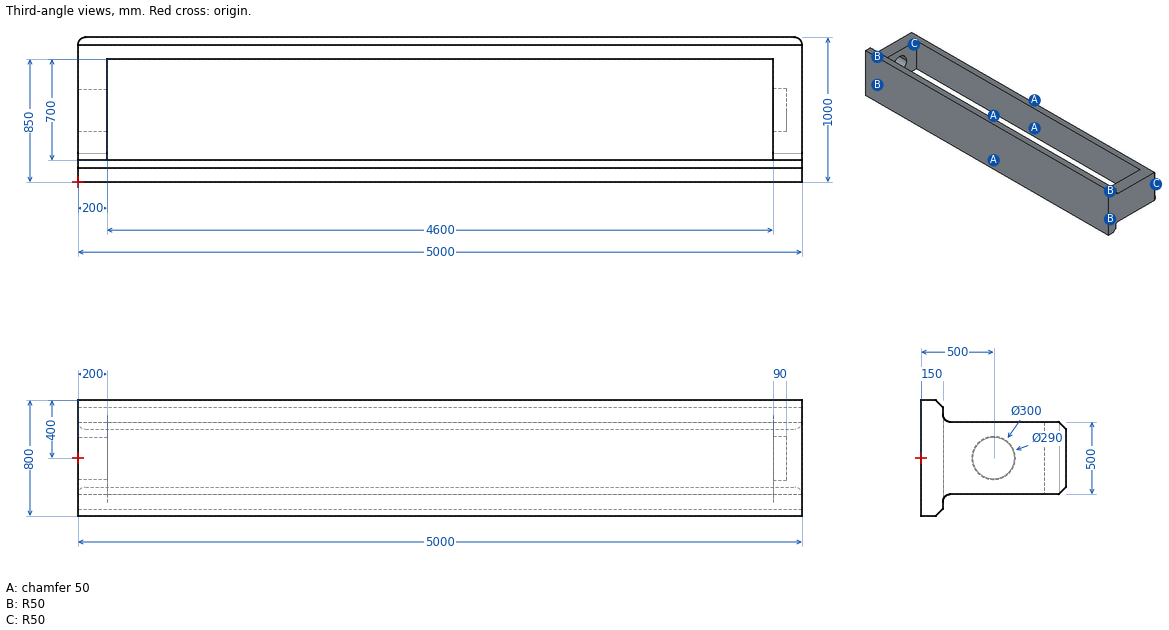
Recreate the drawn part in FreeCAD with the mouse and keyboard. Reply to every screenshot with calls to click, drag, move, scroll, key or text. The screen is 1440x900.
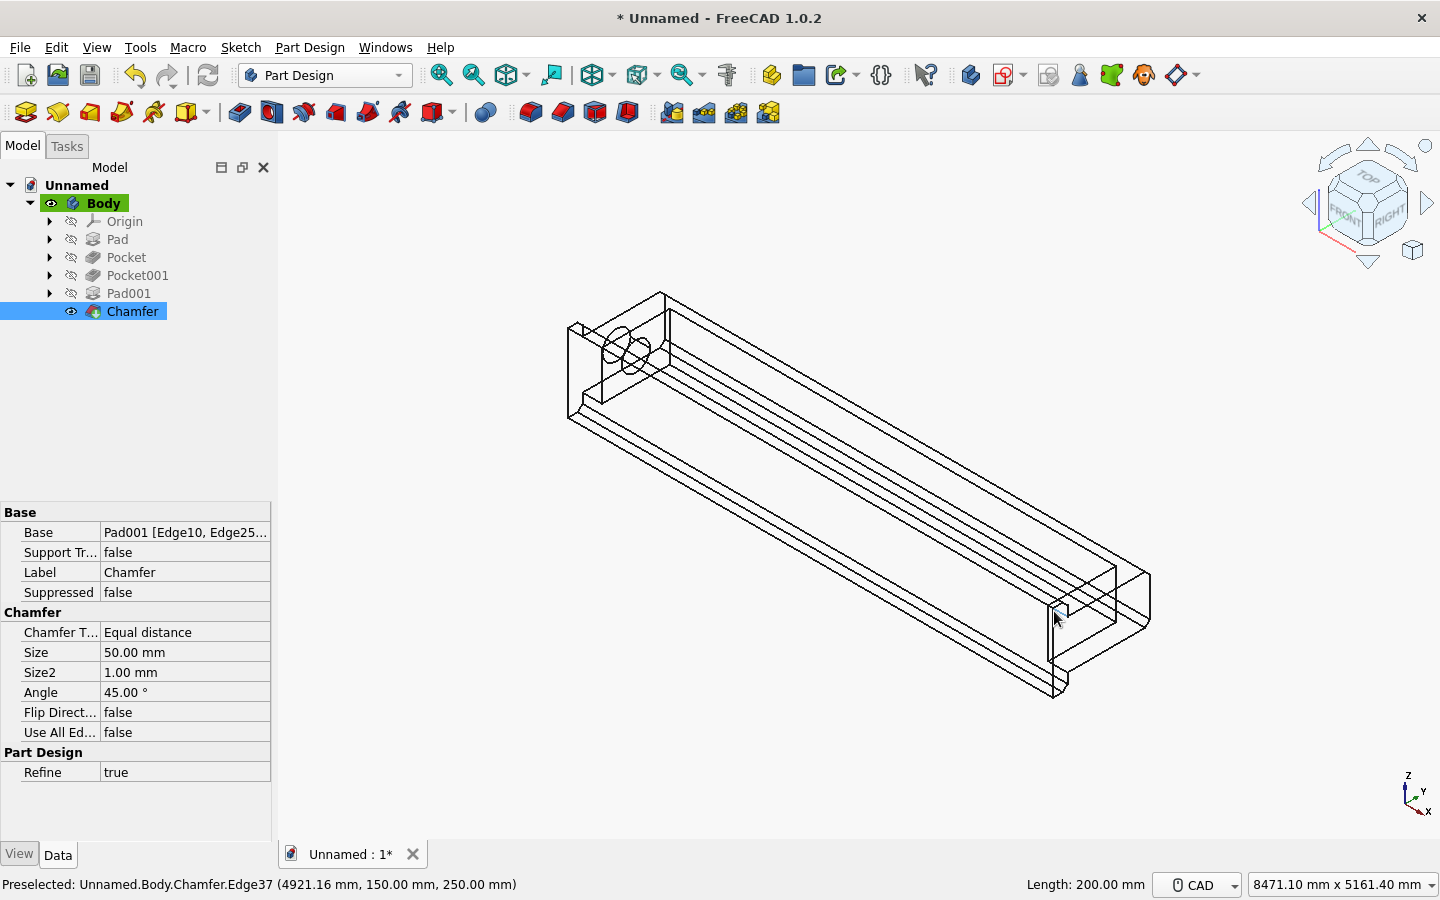
click(1060, 667, ctrl)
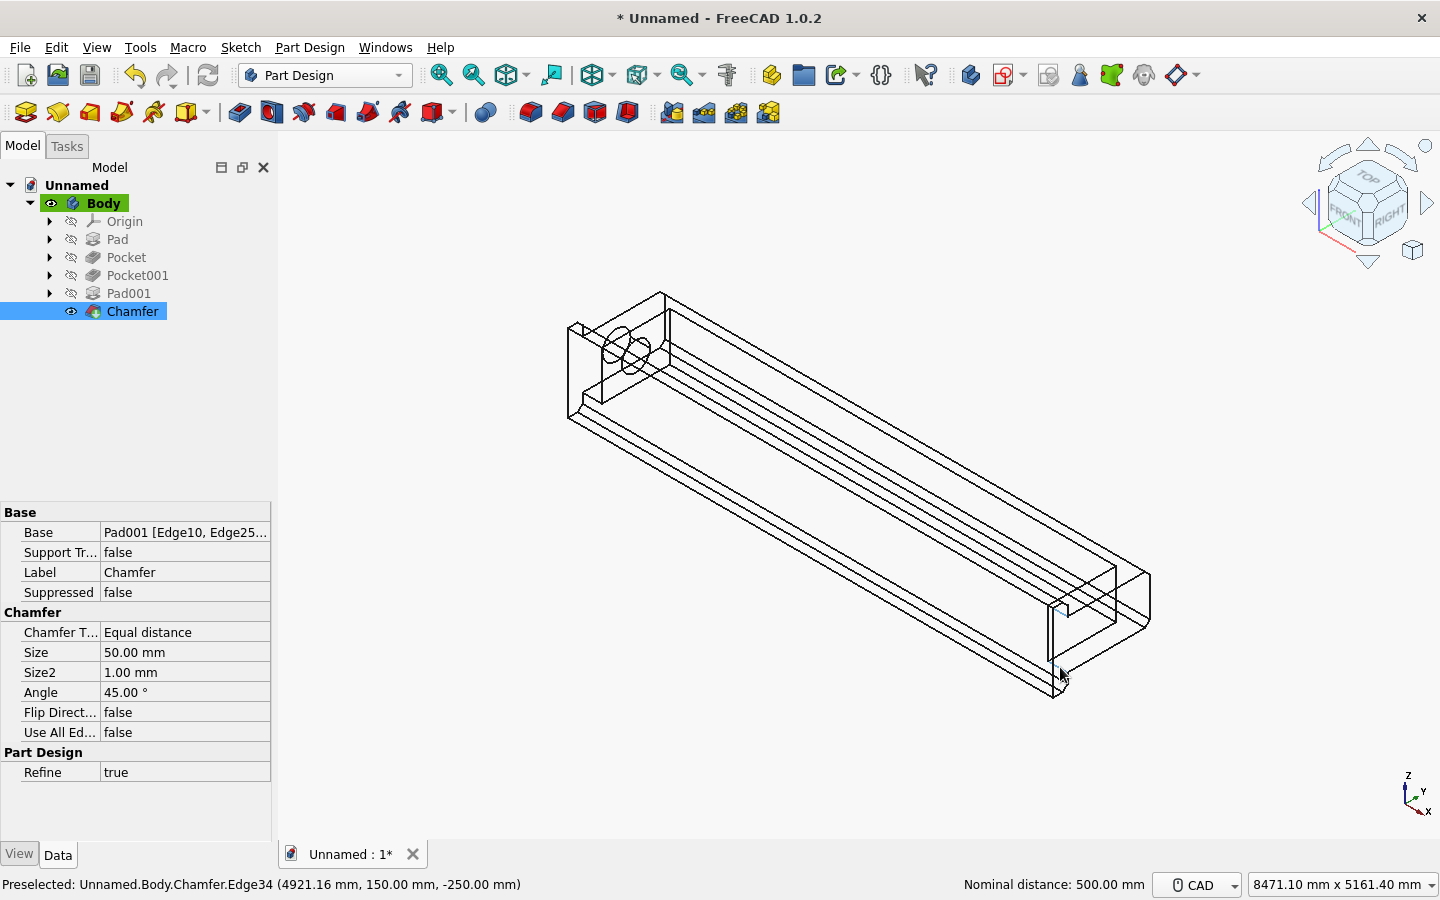
click(592, 397, ctrl)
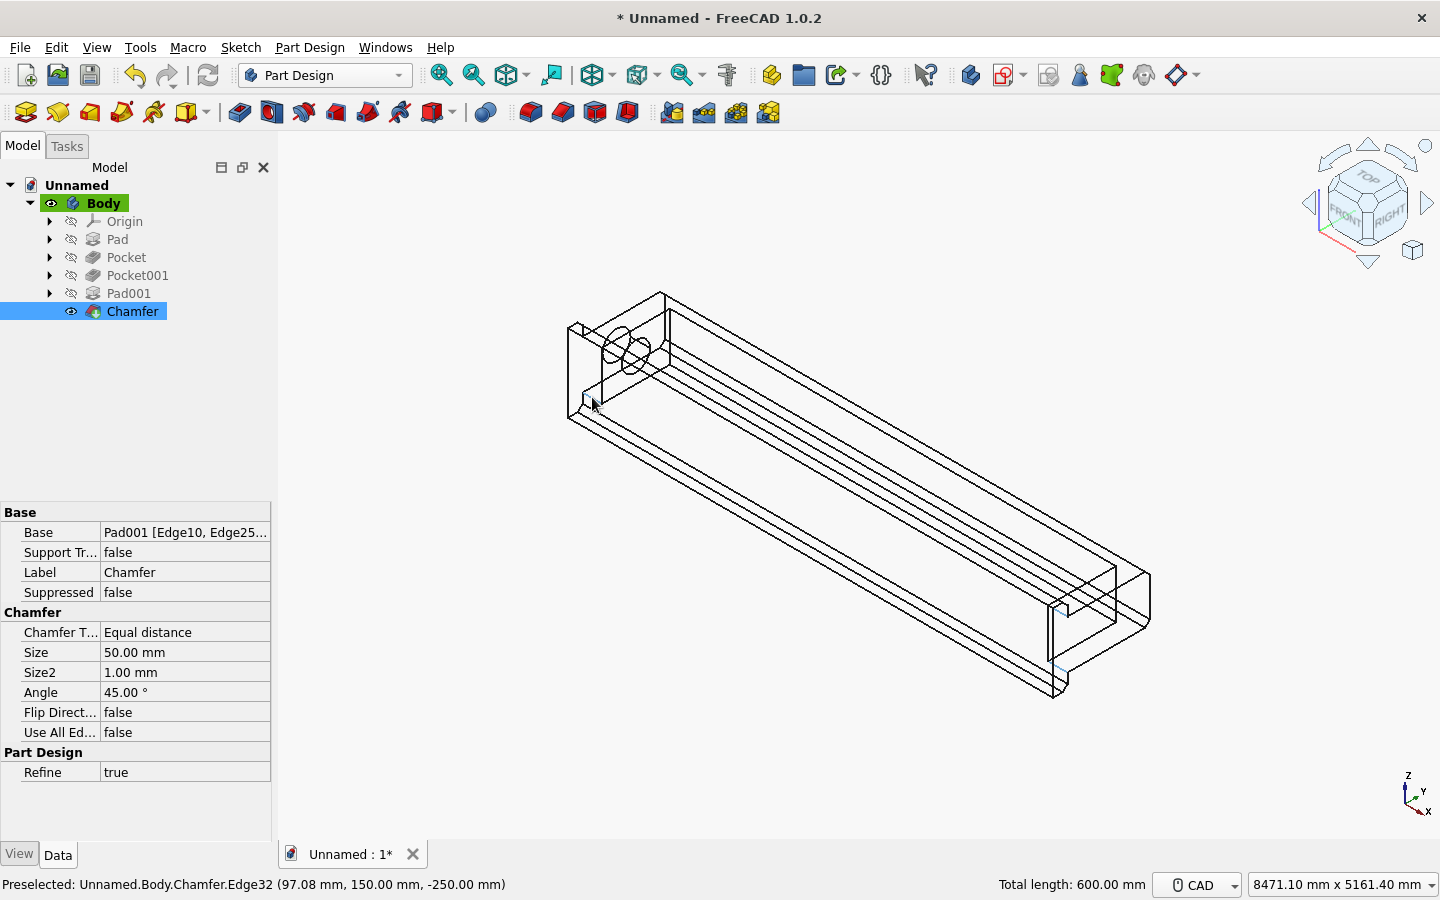
key(2)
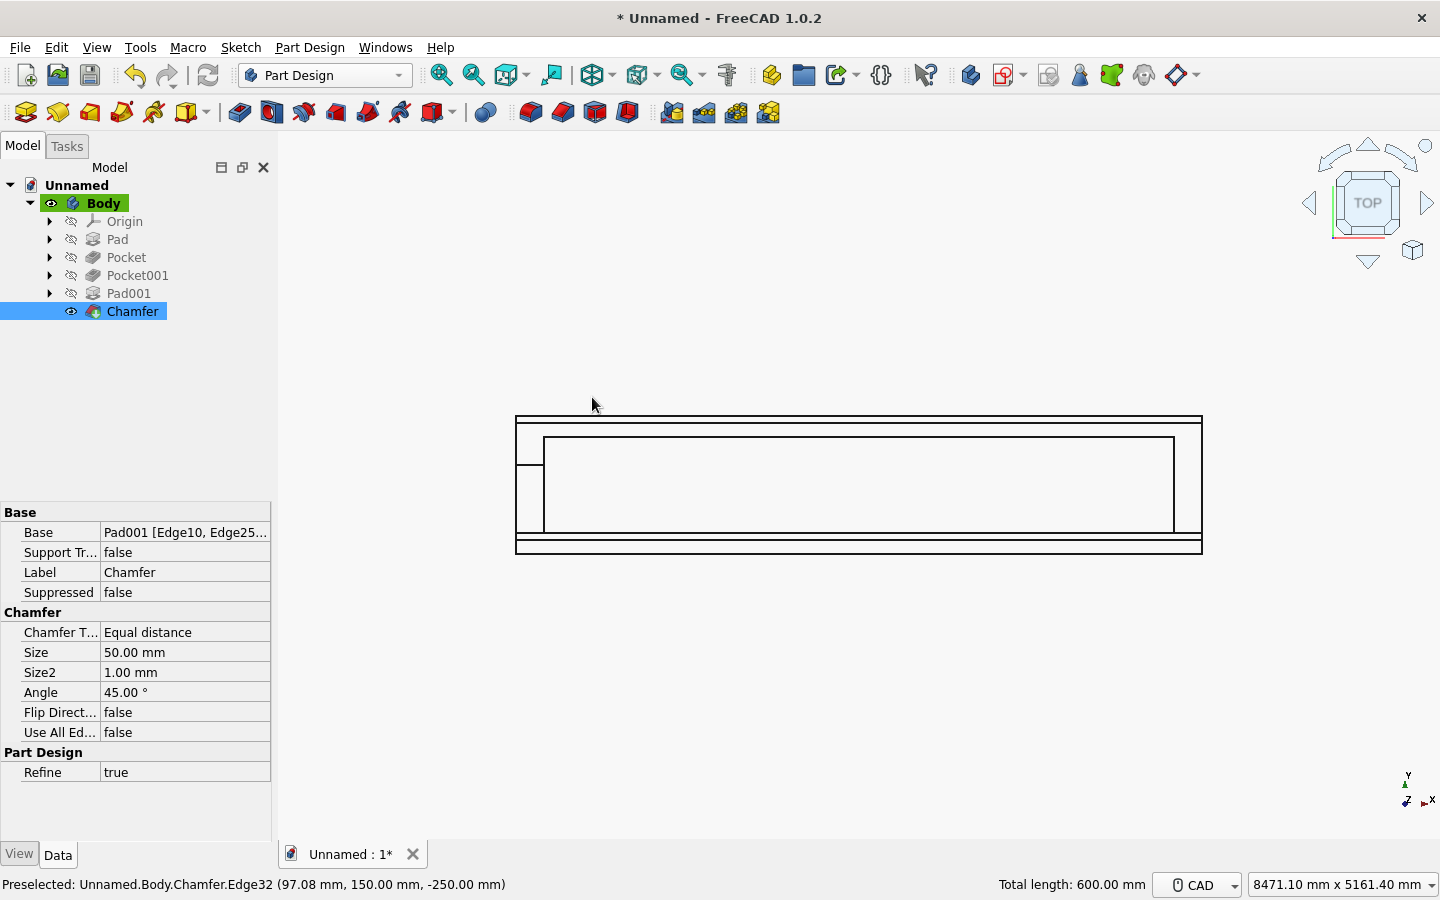
key(1)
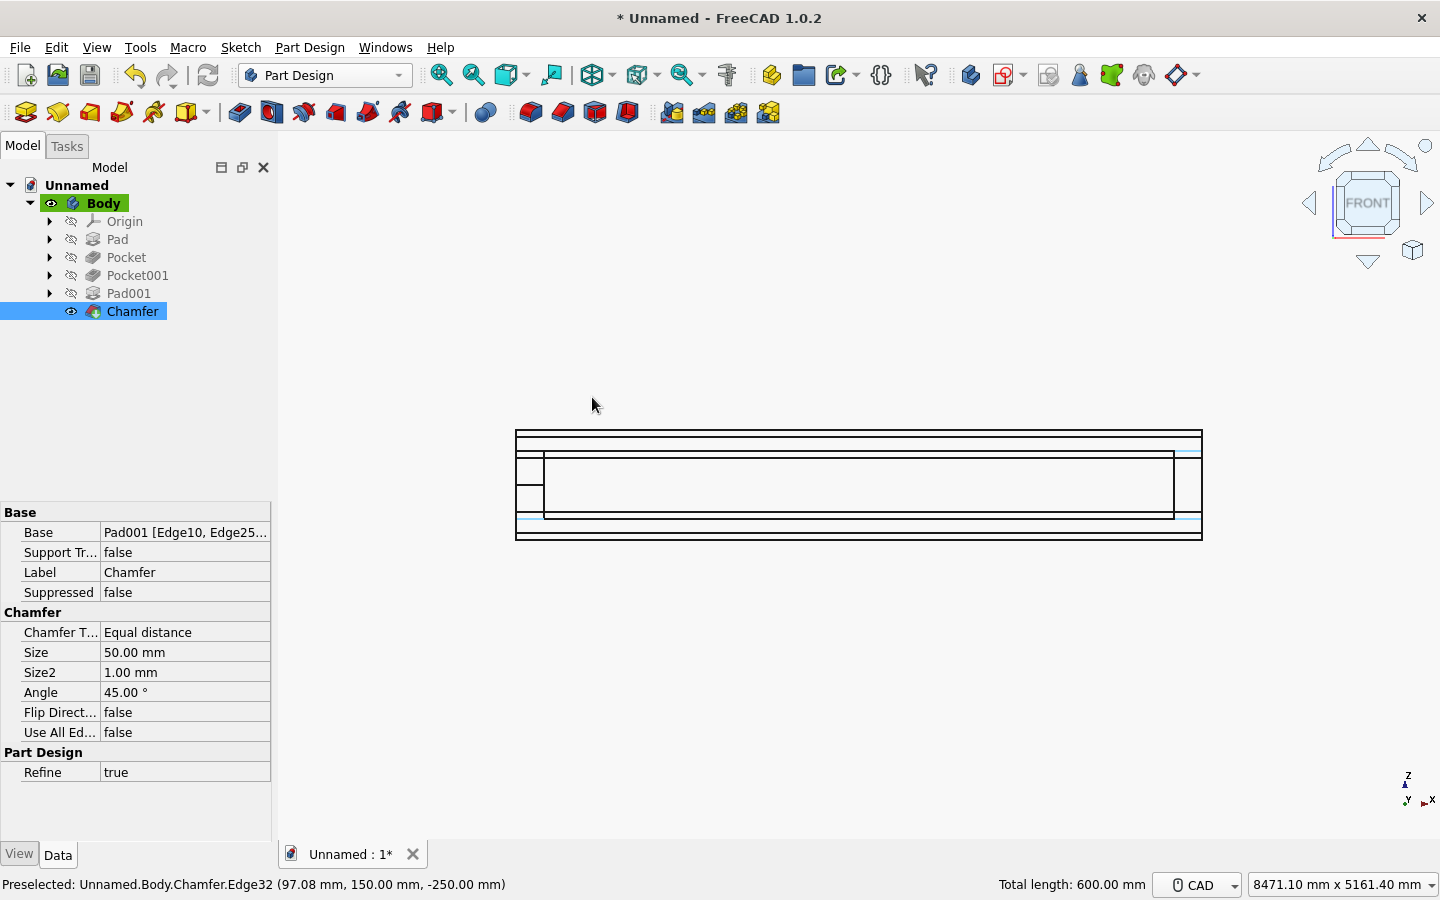
click(530, 450, ctrl)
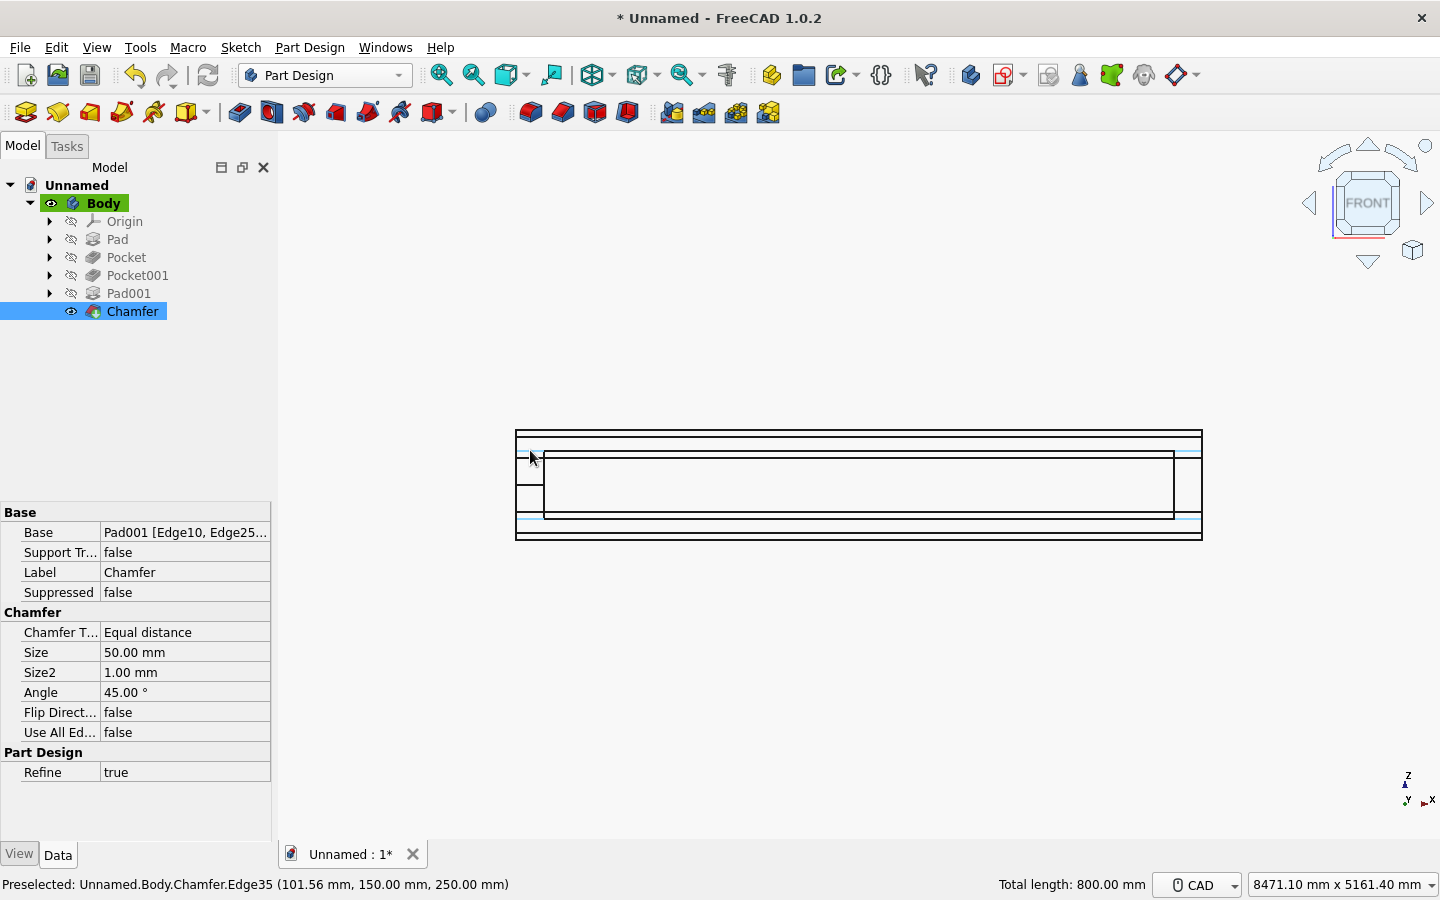
key(v)
key(1)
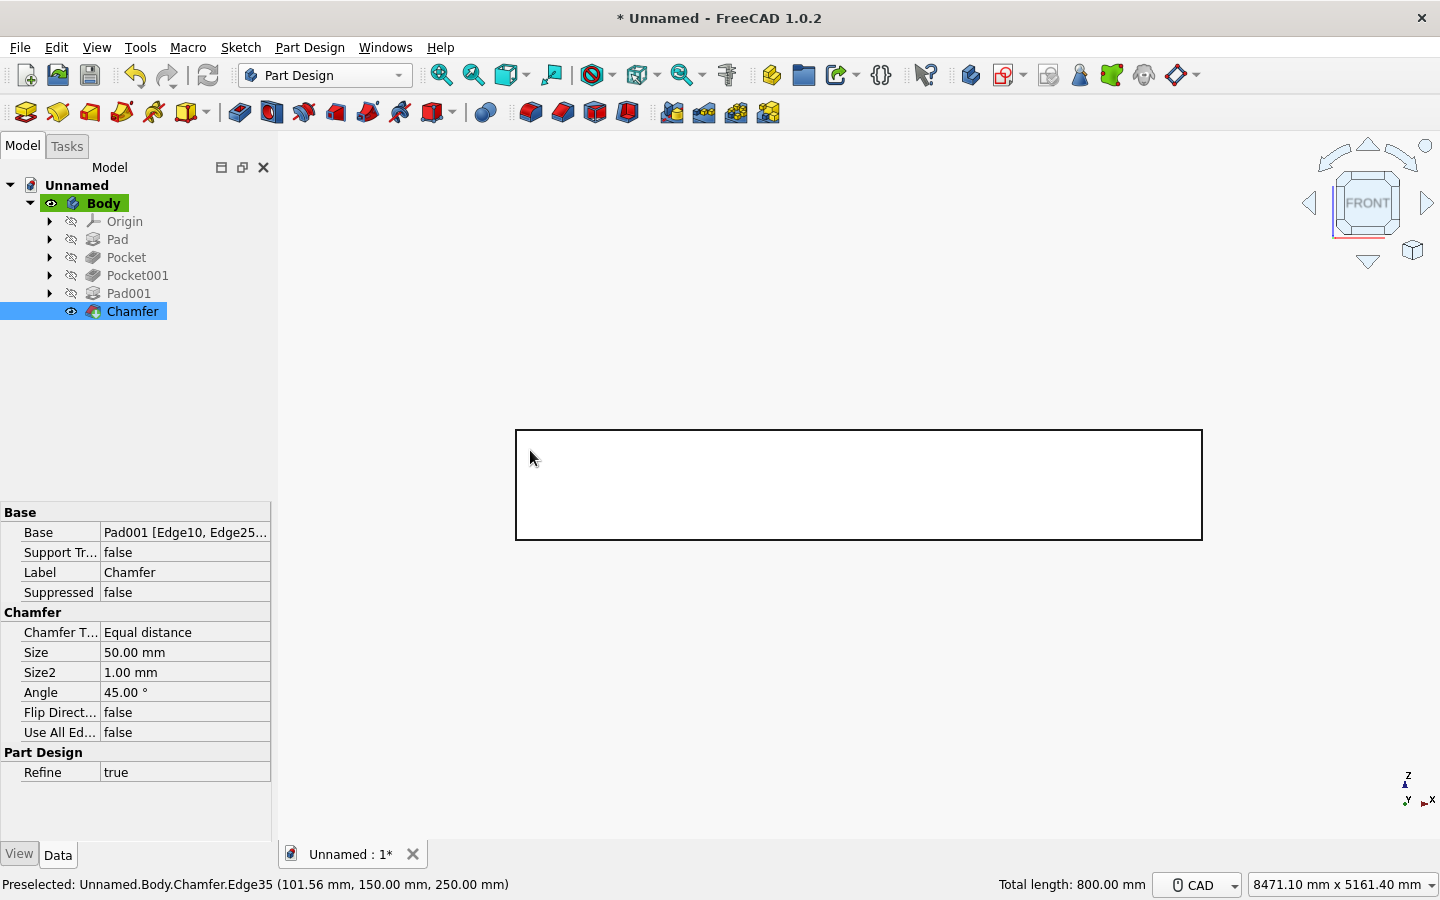
click(532, 112)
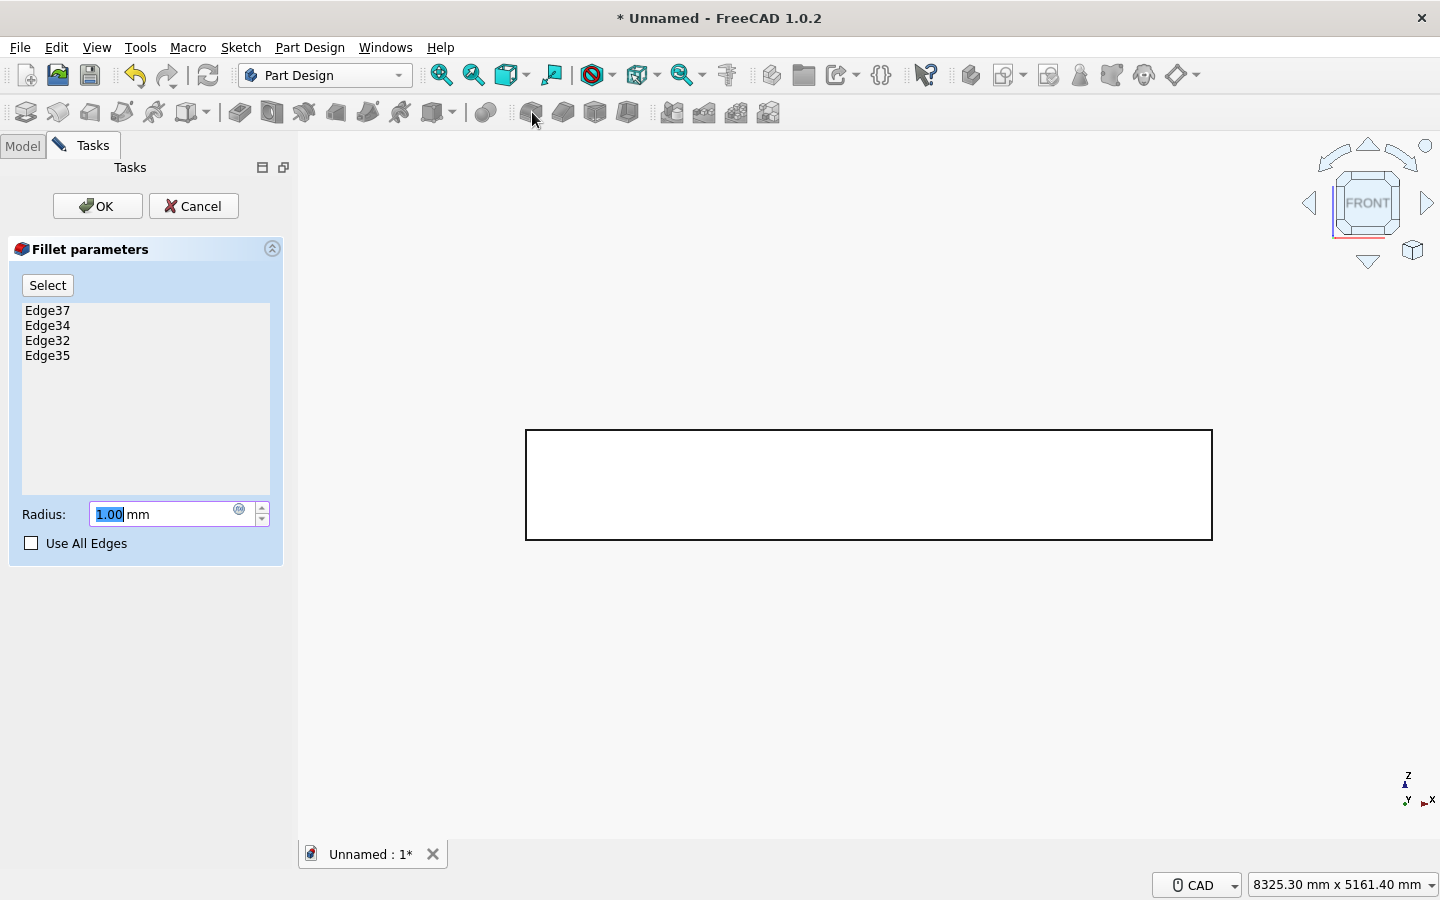
text(50)
key(Tab)